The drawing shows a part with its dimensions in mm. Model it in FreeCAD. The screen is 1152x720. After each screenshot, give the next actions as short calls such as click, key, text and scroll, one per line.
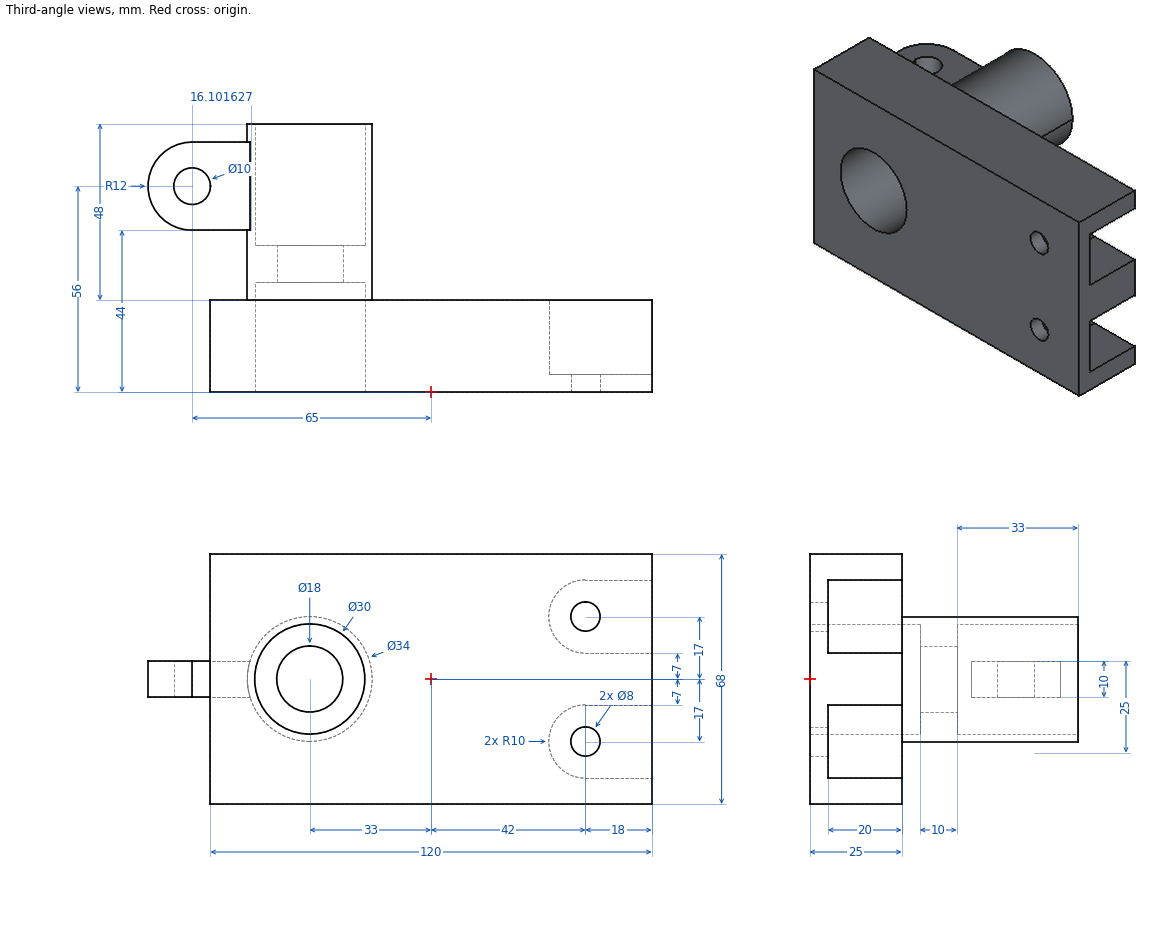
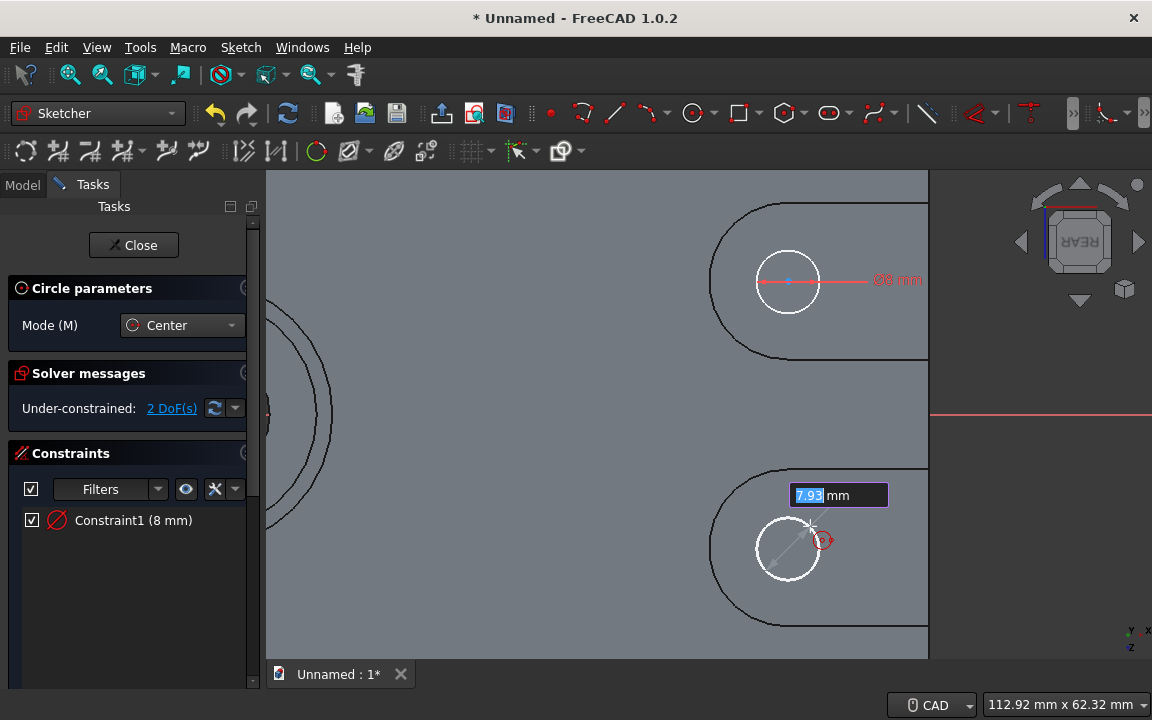
text(8)
key(Return)
key(Escape)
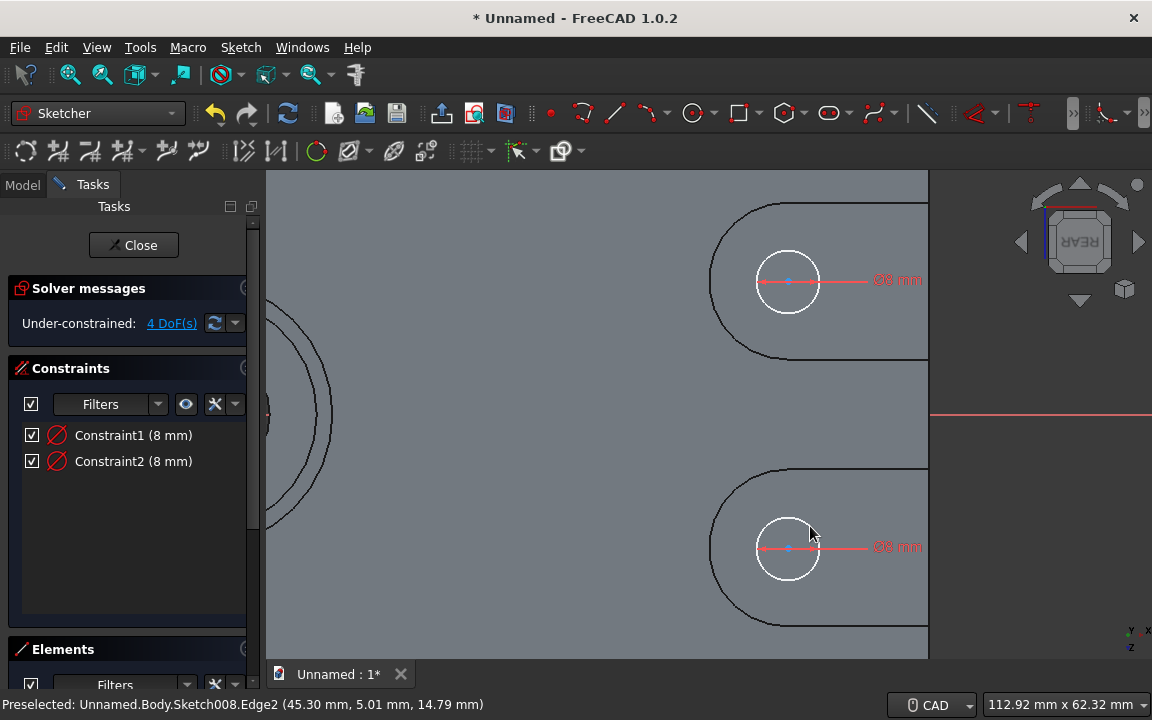
click(974, 114)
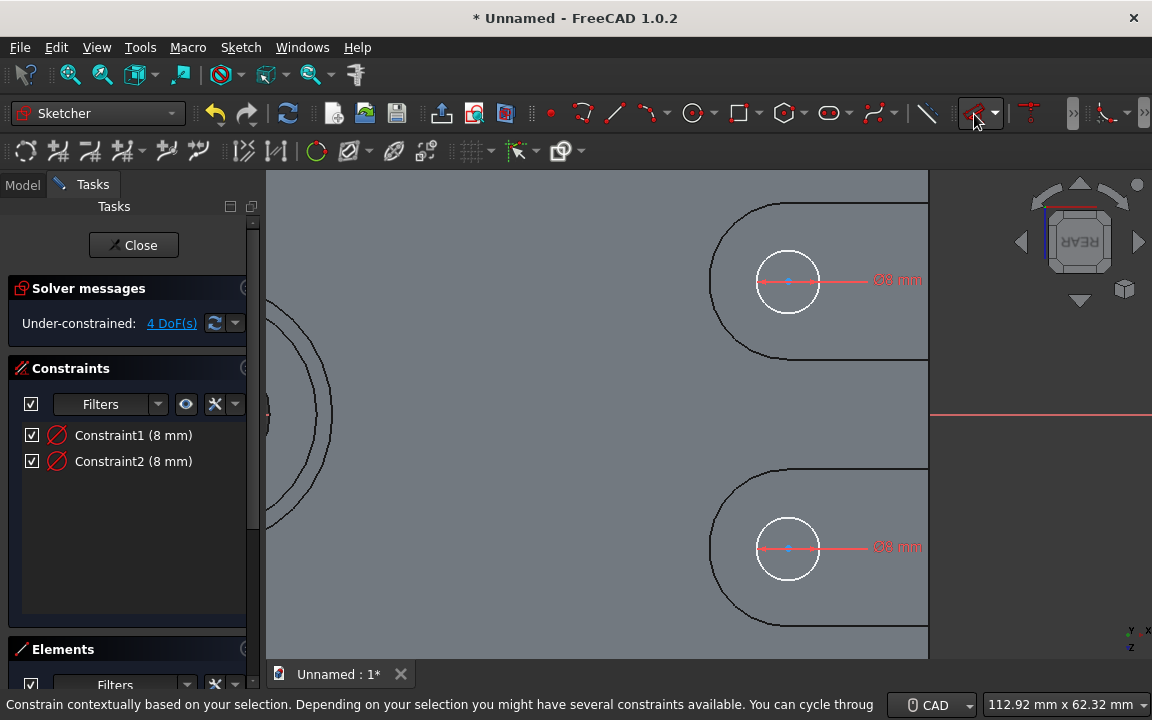
click(788, 282)
click(623, 248)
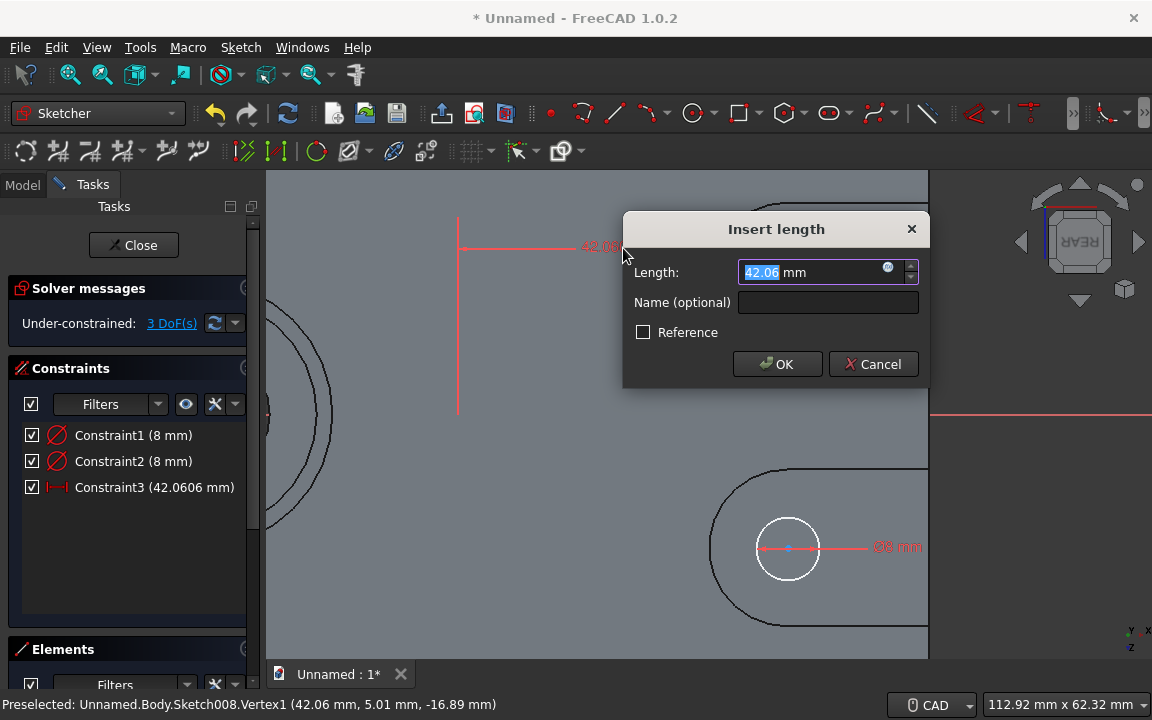
text(42)
key(Return)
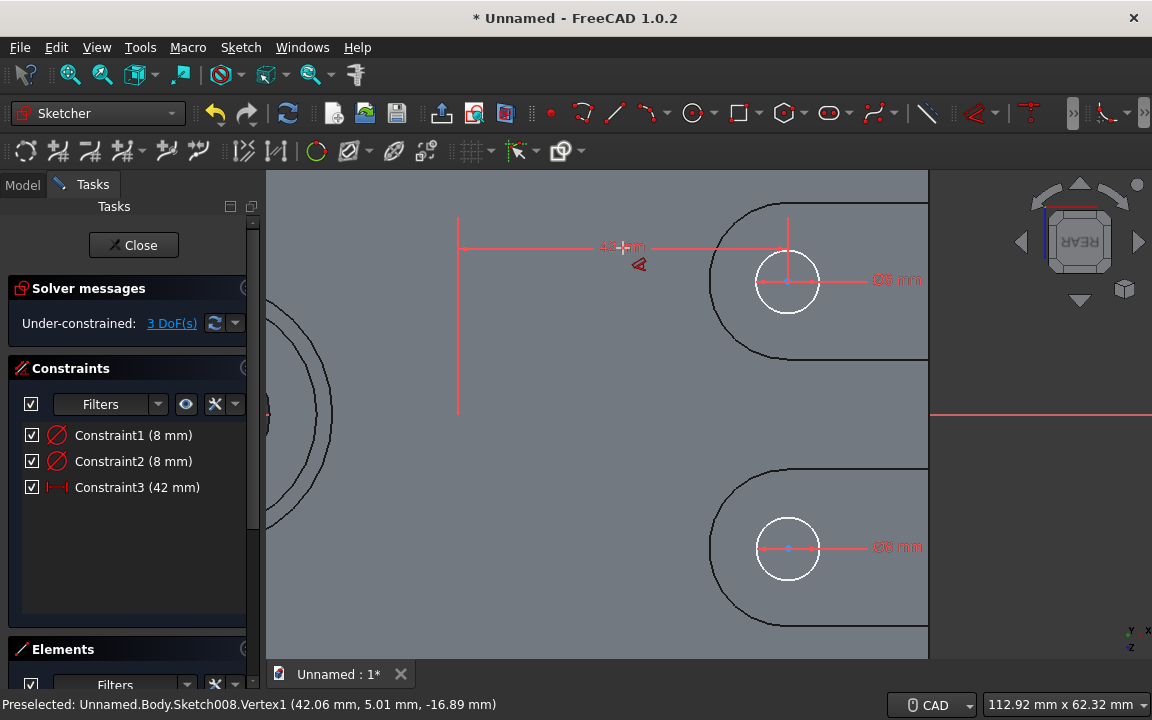
click(788, 282)
click(424, 348)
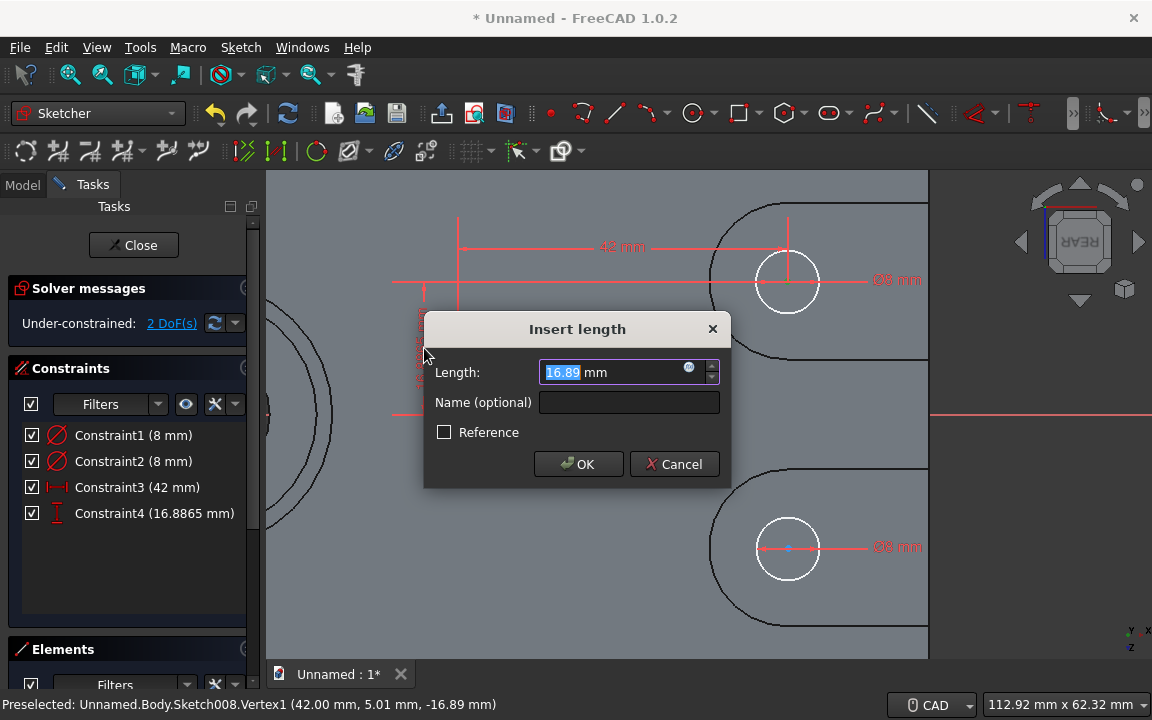
text(17)
key(Return)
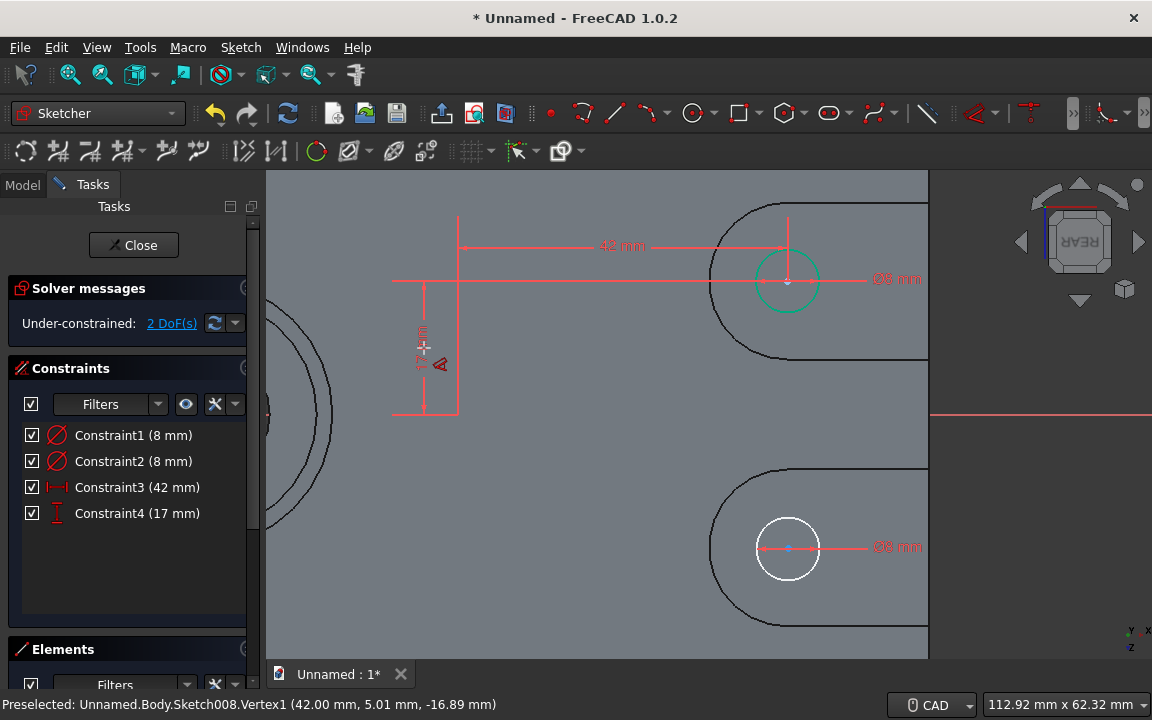
click(788, 549)
click(623, 583)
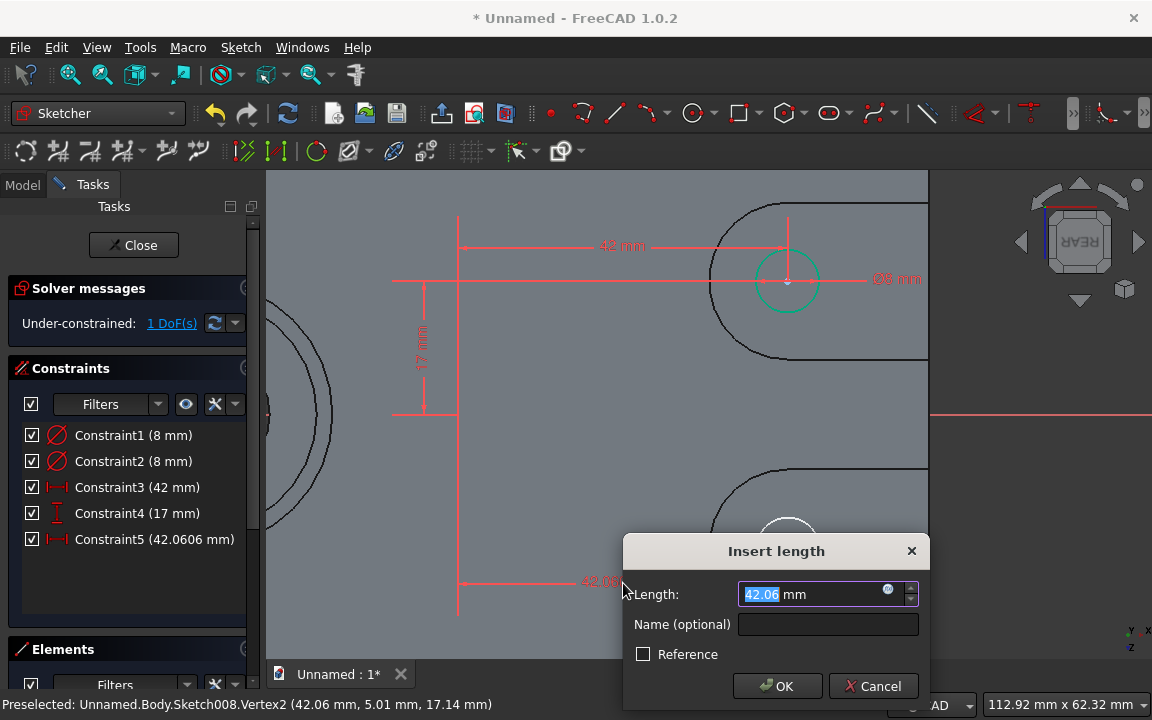
text(42)
key(Return)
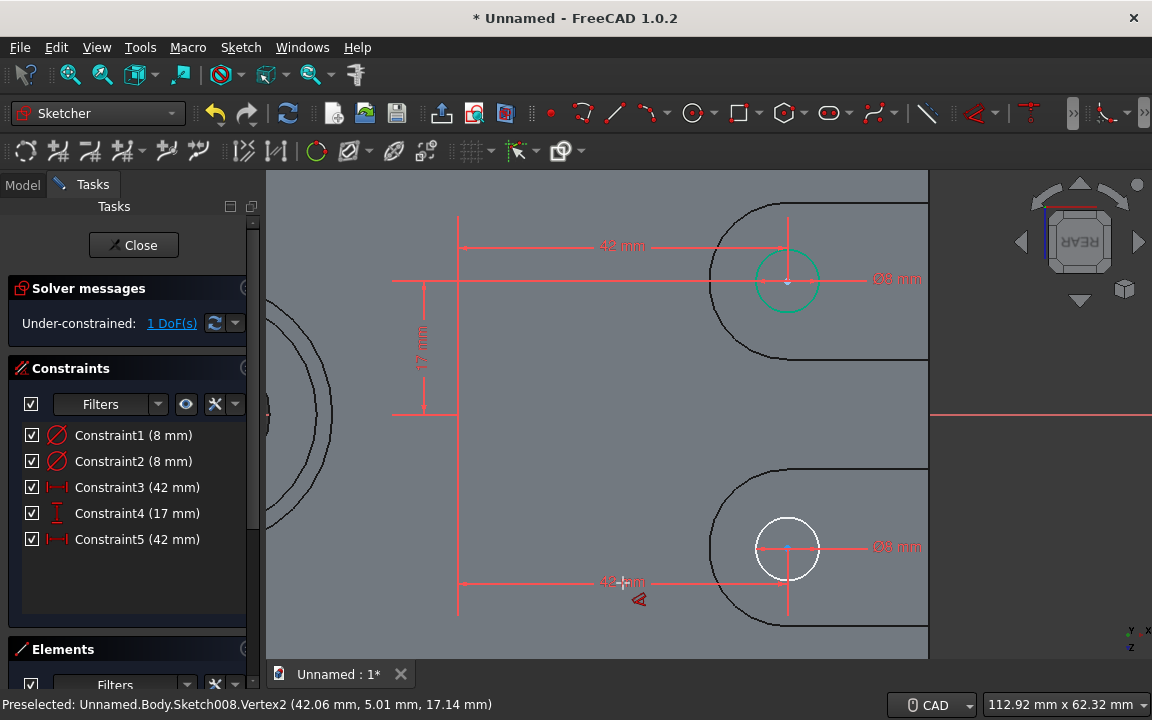
click(788, 549)
click(424, 482)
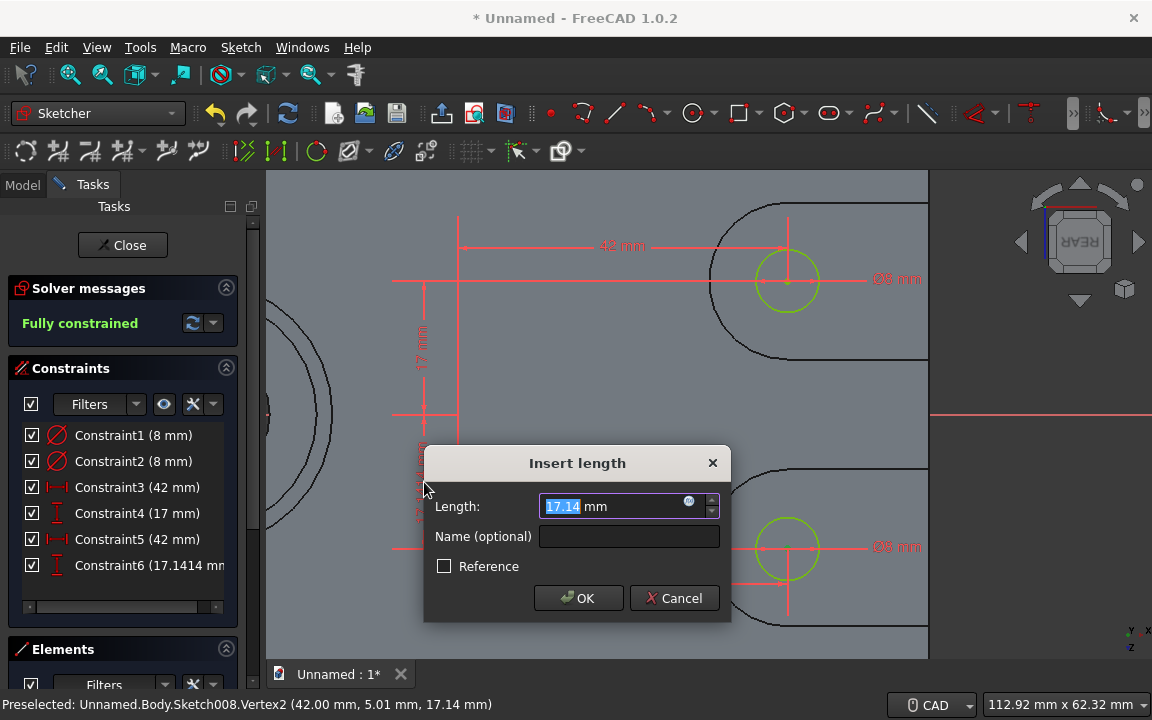
text(17)
key(Return)
key(Escape)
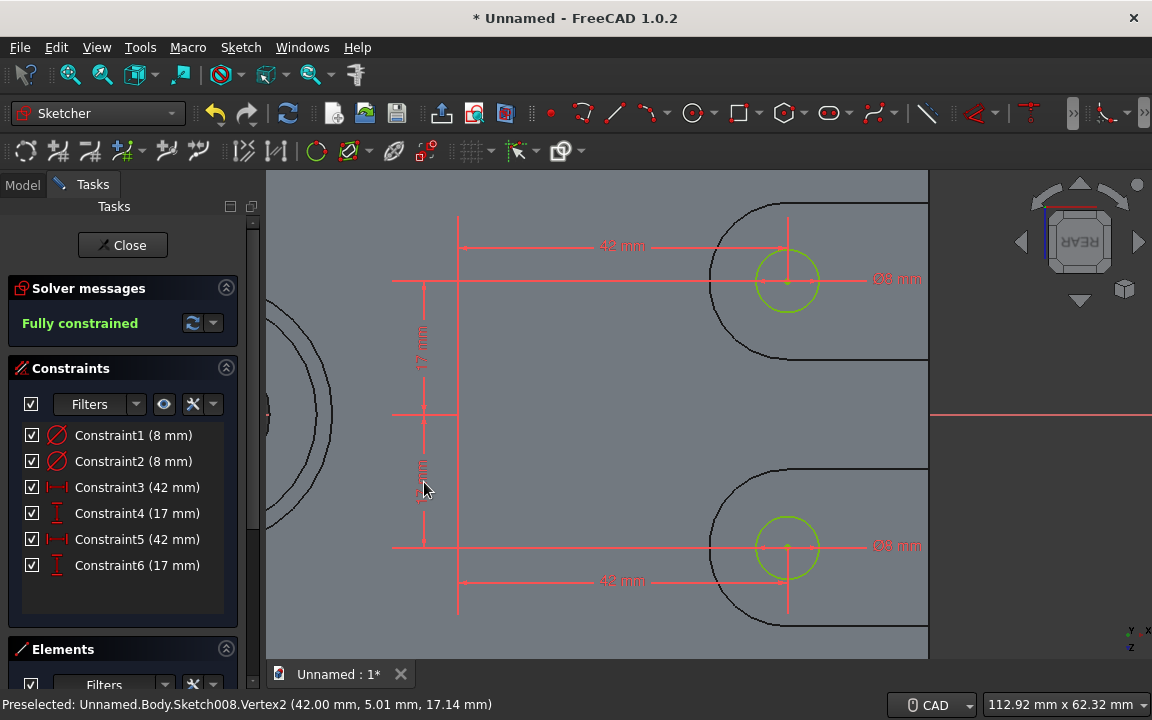
click(123, 245)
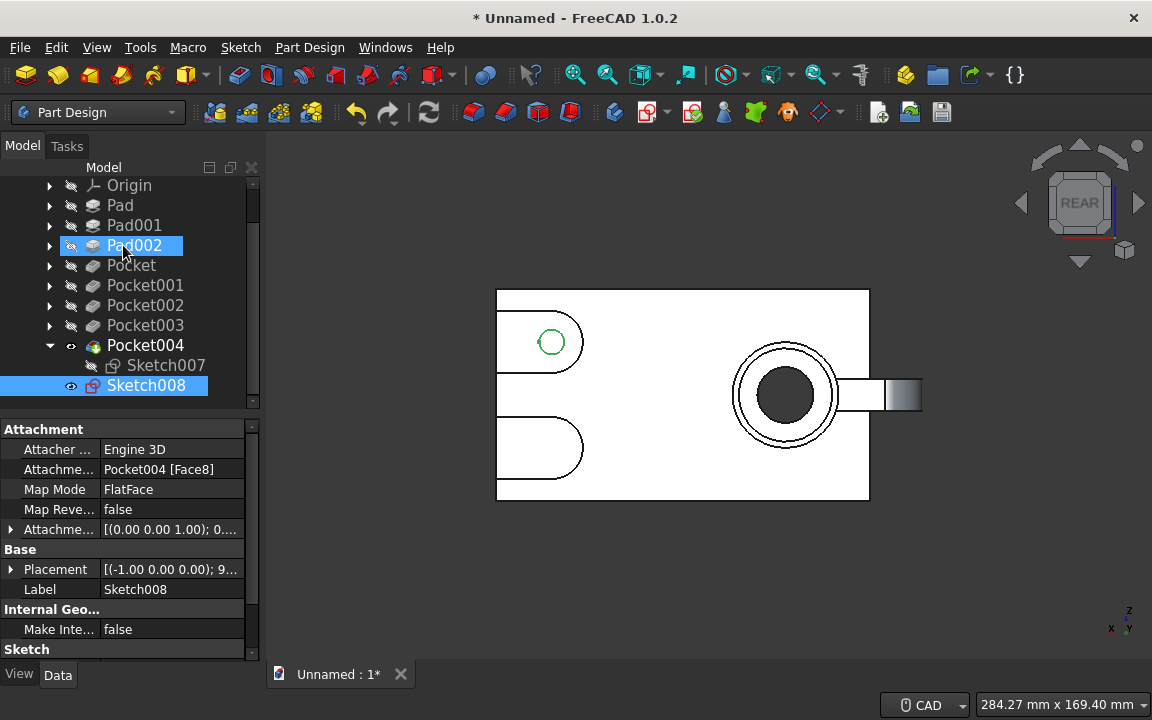
click(240, 76)